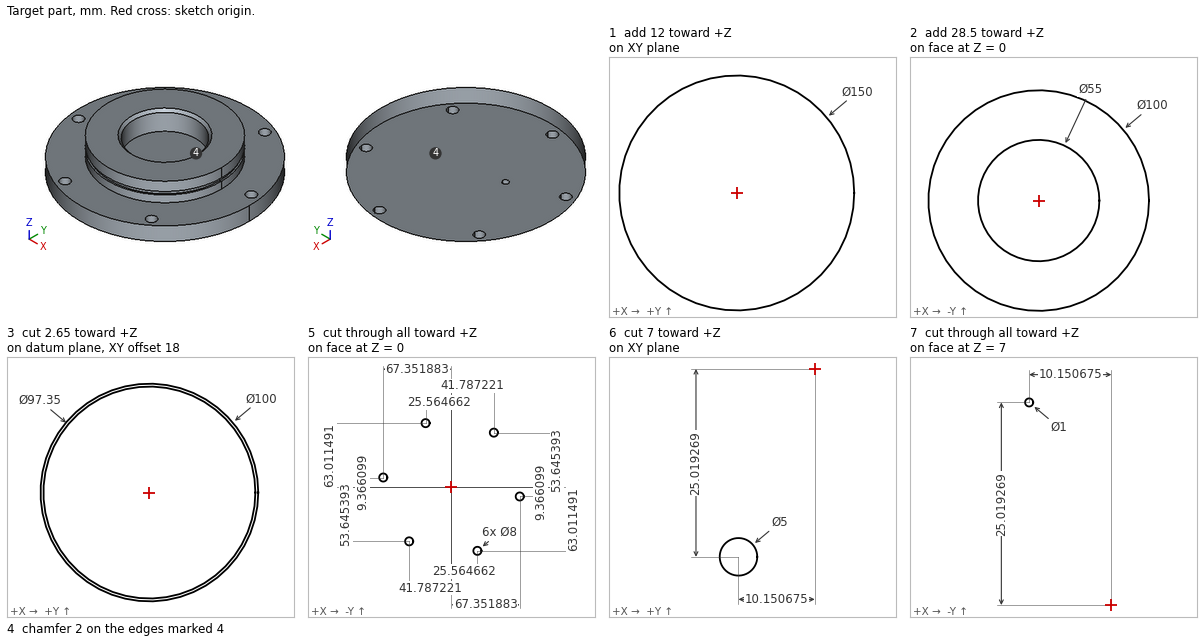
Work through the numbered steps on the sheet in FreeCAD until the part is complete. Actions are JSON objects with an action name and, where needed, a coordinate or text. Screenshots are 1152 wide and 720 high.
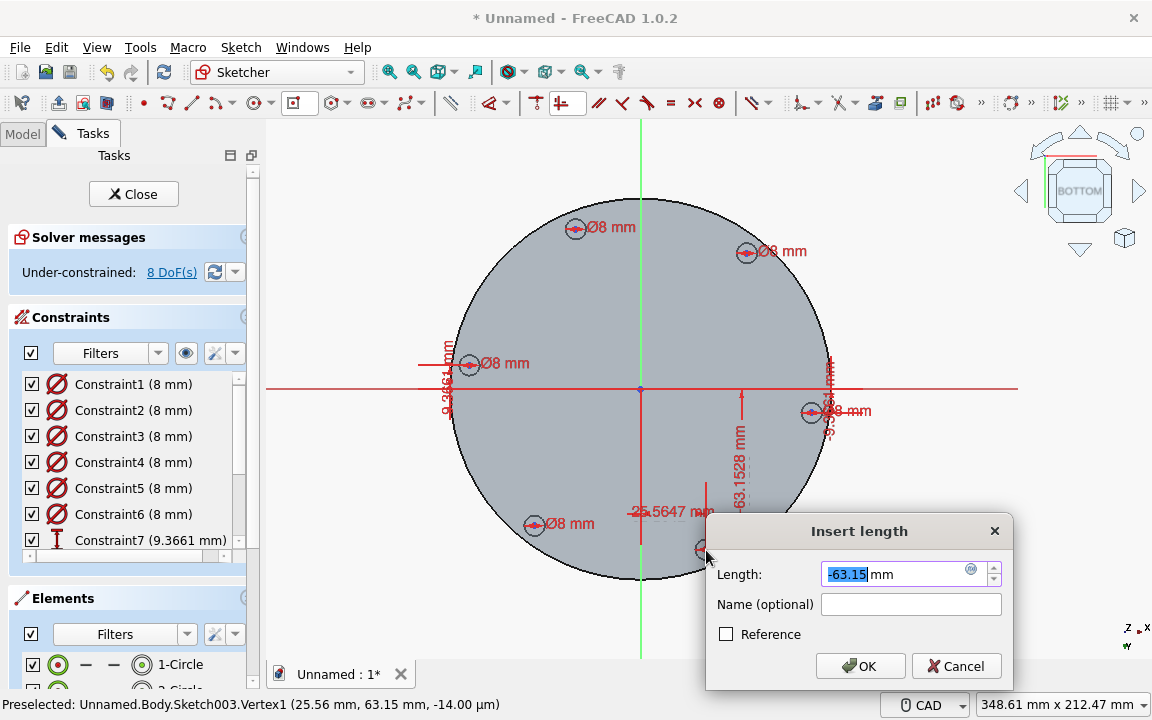
{"action": "type", "text": "-63.011491"}
{"action": "key", "text": "Return"}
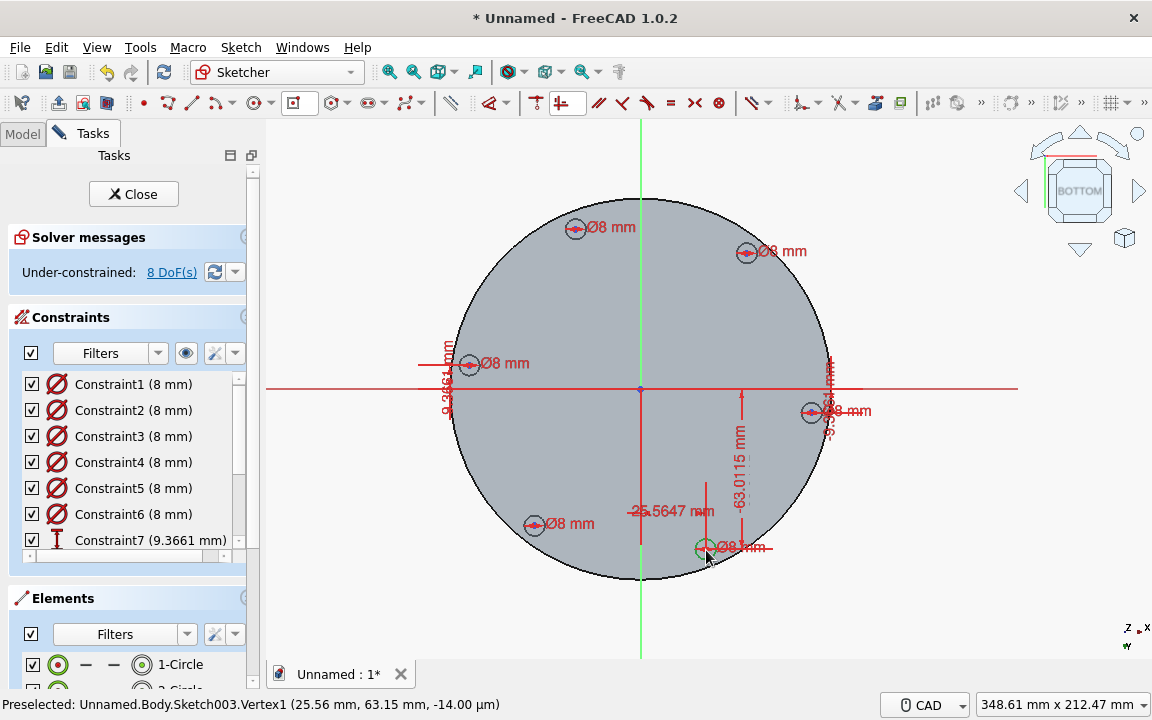
{"action": "left_click", "coordinate": [535, 526]}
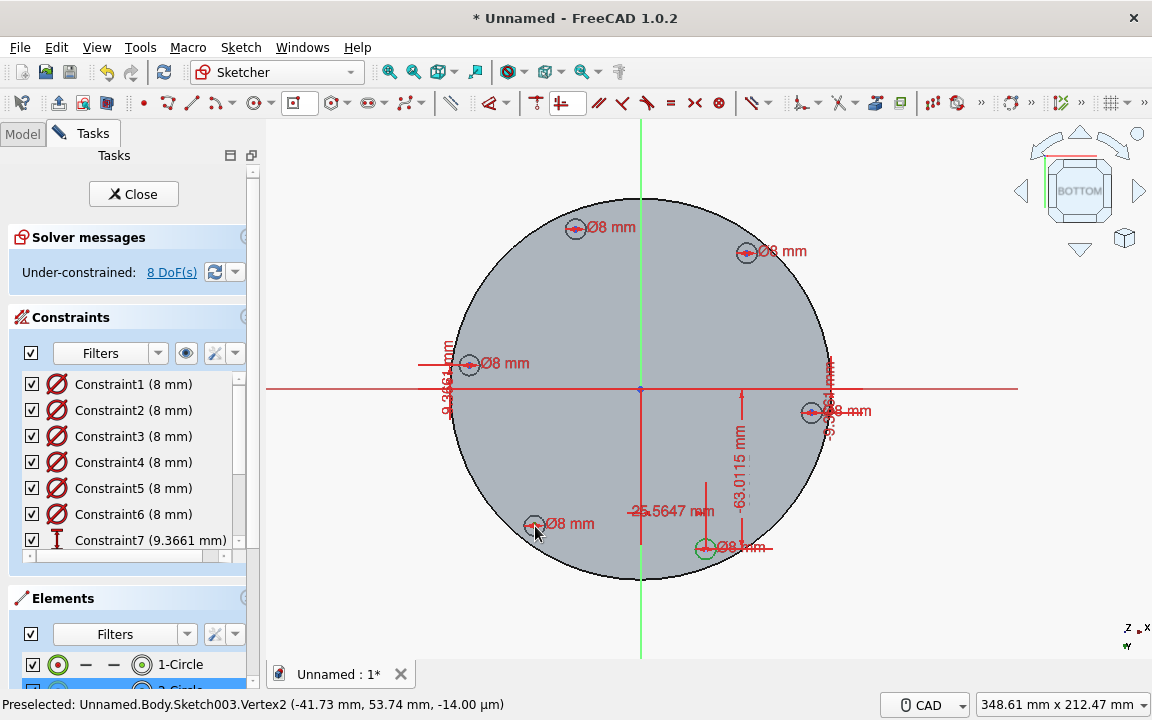
{"action": "left_click", "coordinate": [508, 104]}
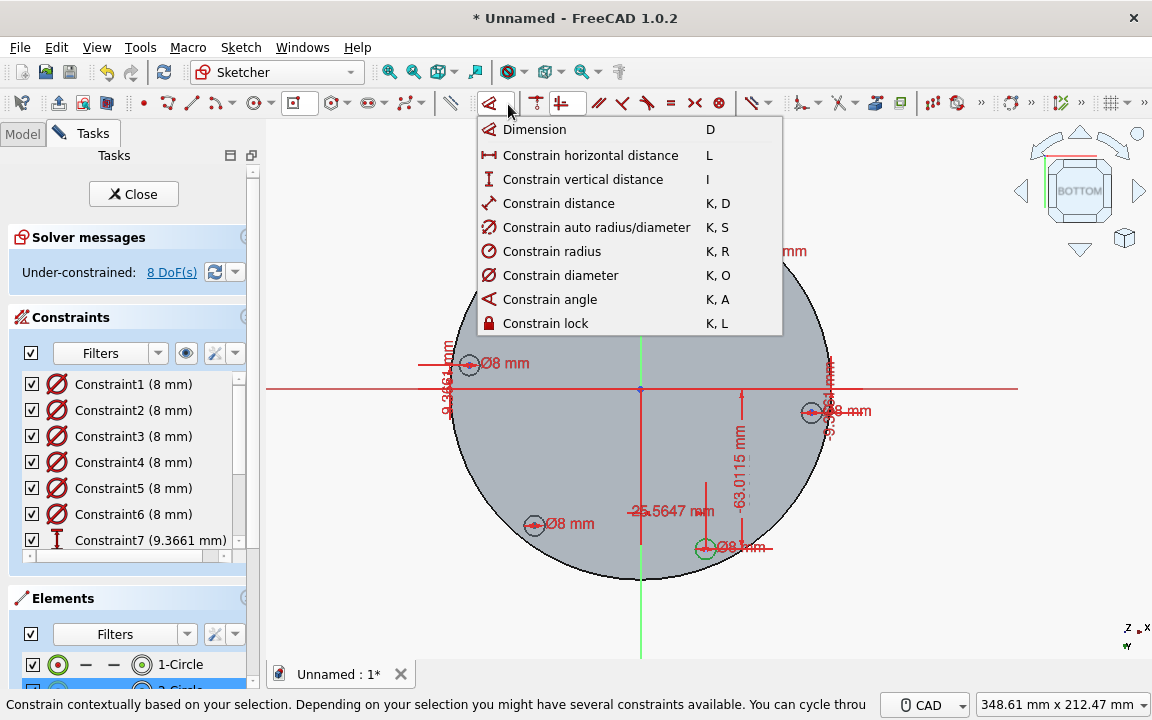
{"action": "left_click", "coordinate": [630, 155]}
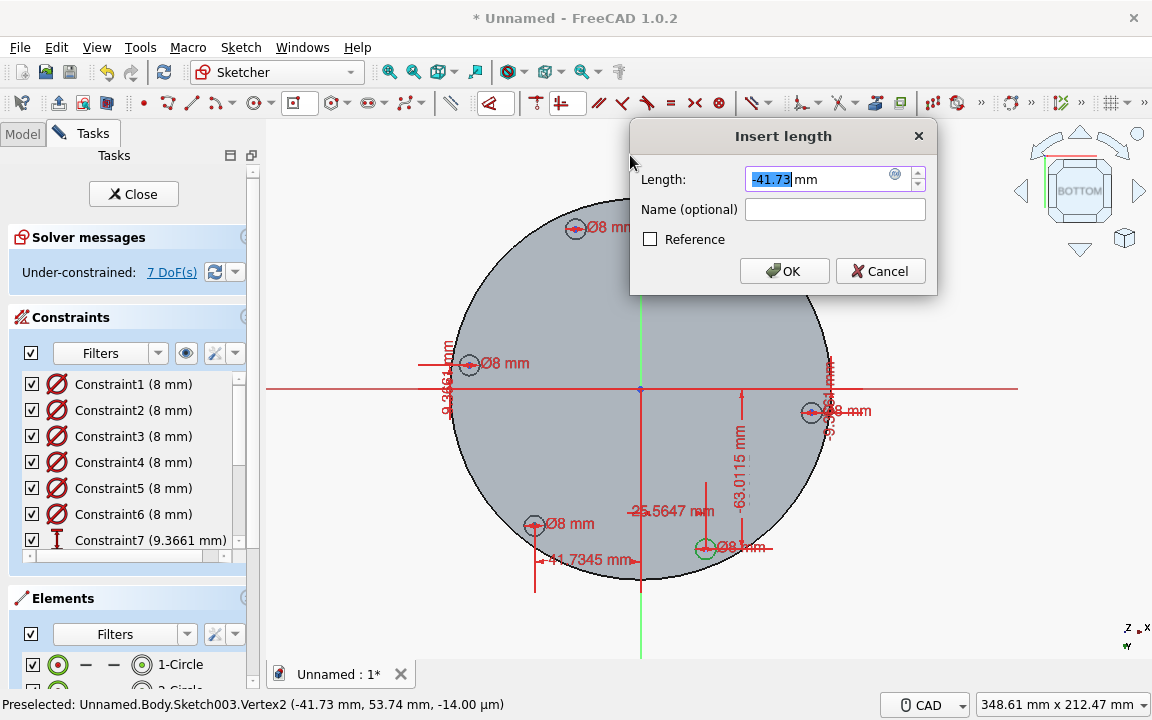
{"action": "type", "text": "-41.787221"}
{"action": "key", "text": "Return"}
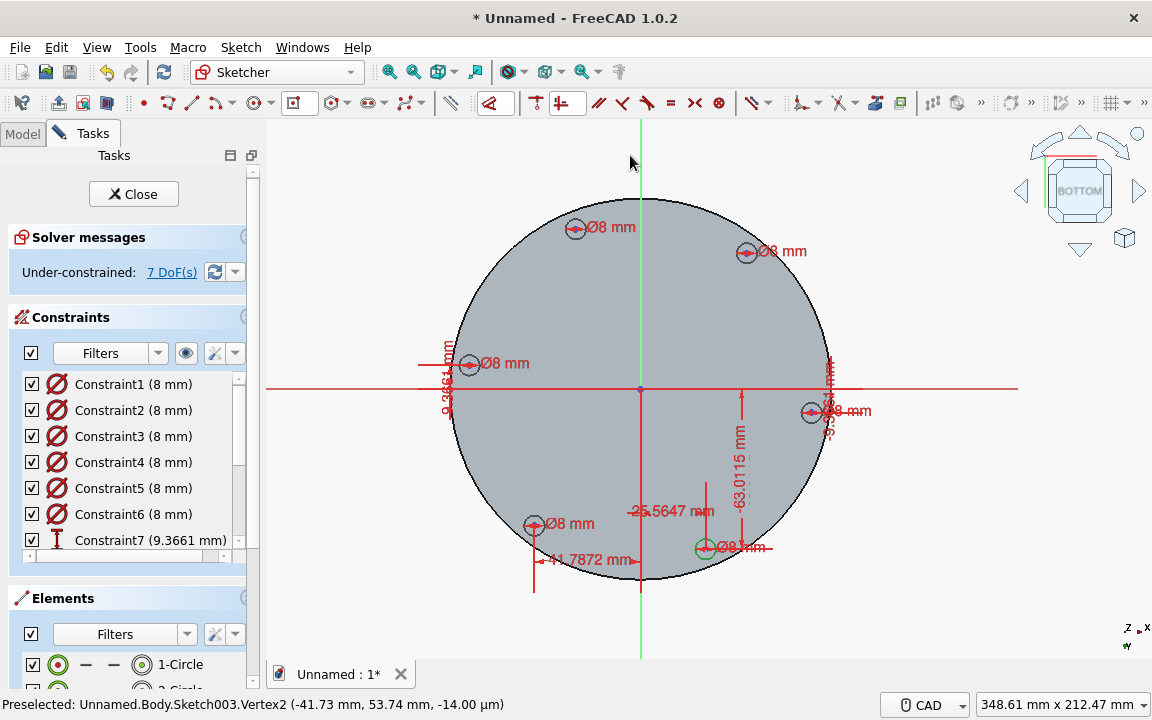
{"action": "left_click", "coordinate": [534, 526]}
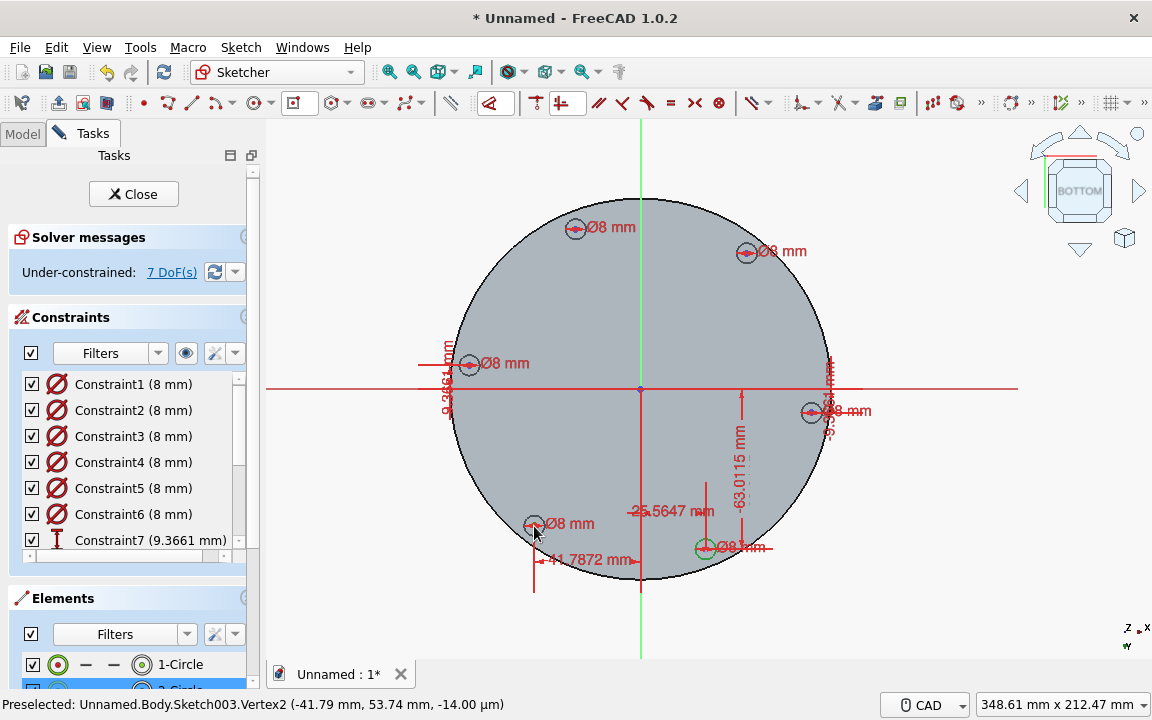
{"action": "key", "text": "i"}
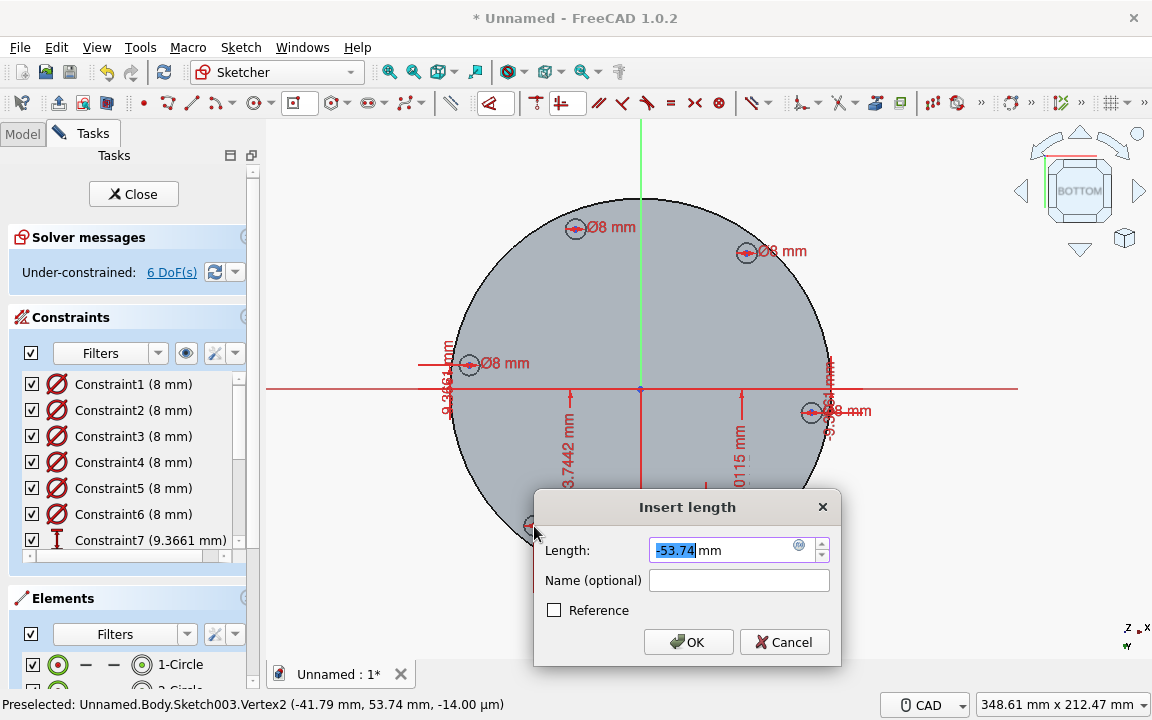
{"action": "type", "text": "-53.645393"}
{"action": "key", "text": "Return"}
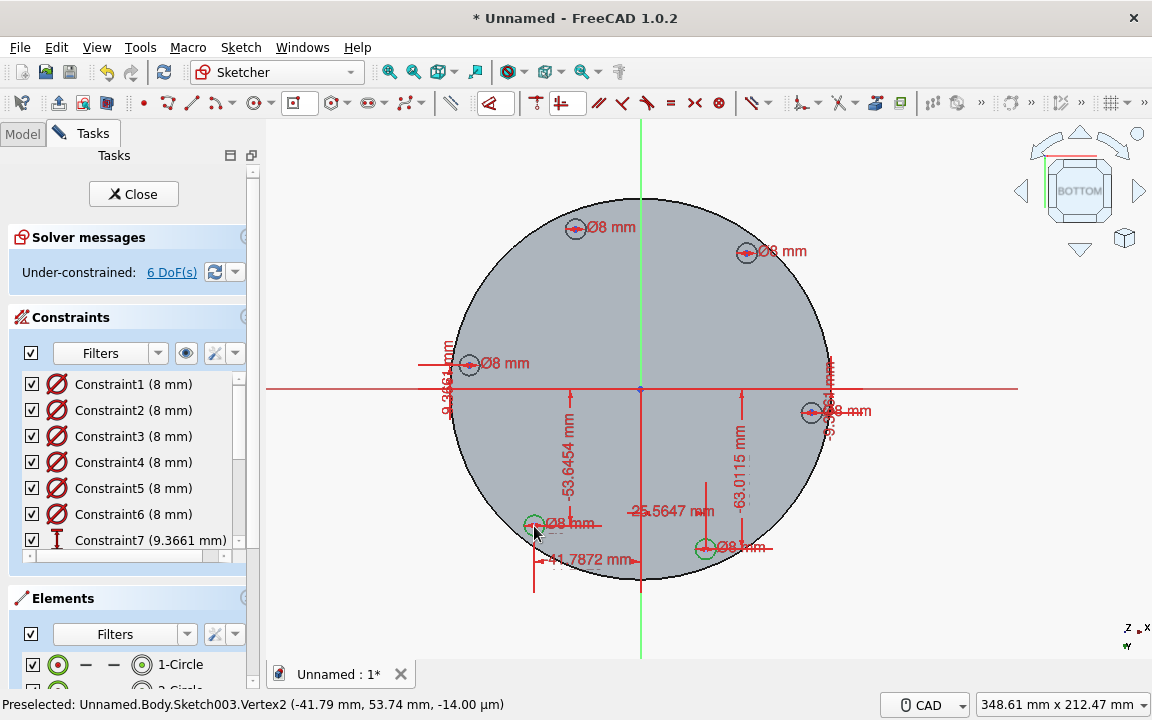
{"action": "left_click", "coordinate": [470, 365]}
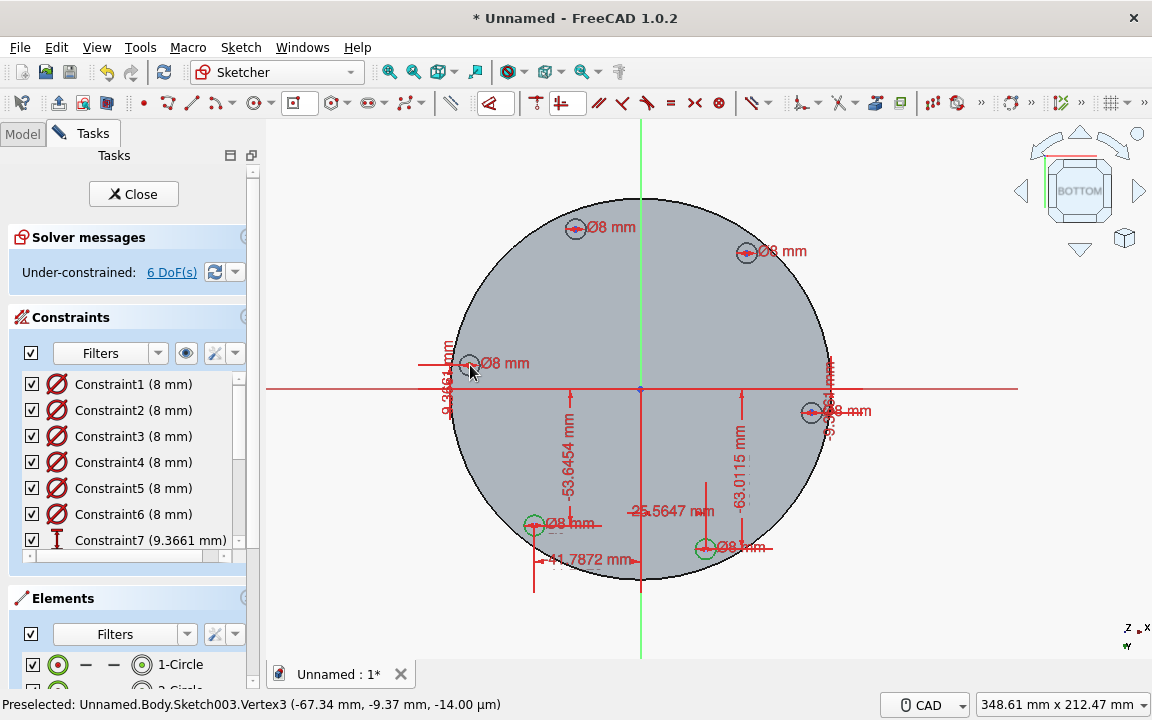
{"action": "left_click", "coordinate": [508, 104]}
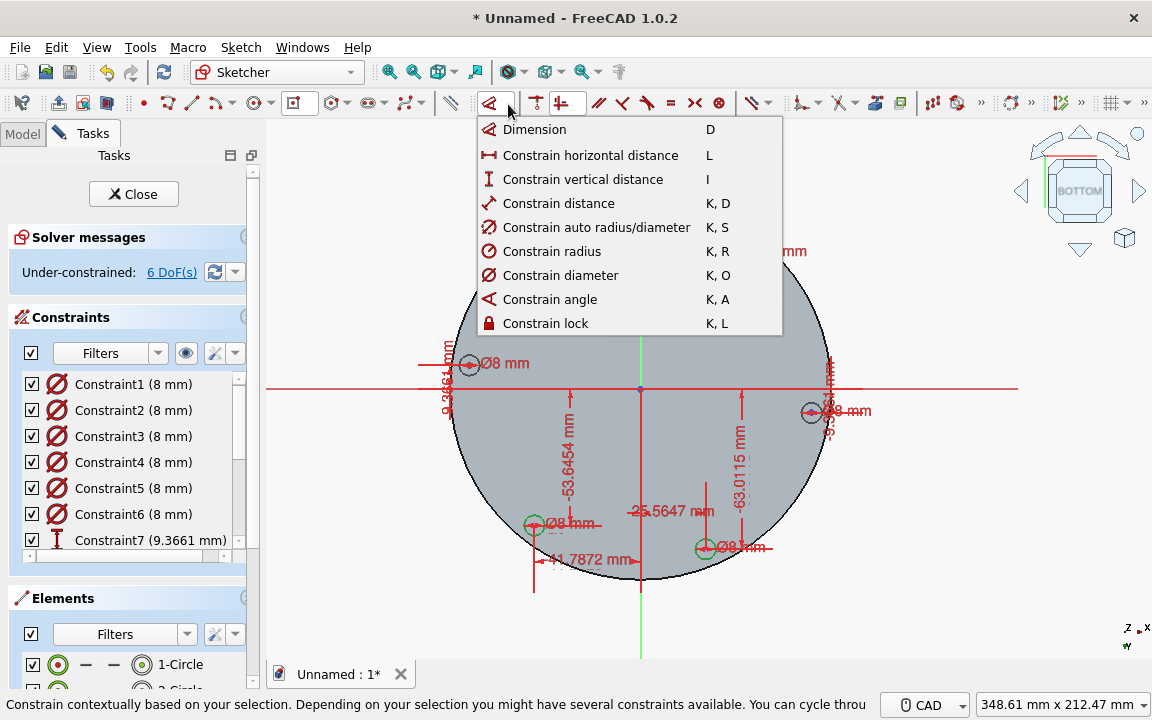
{"action": "left_click", "coordinate": [630, 155]}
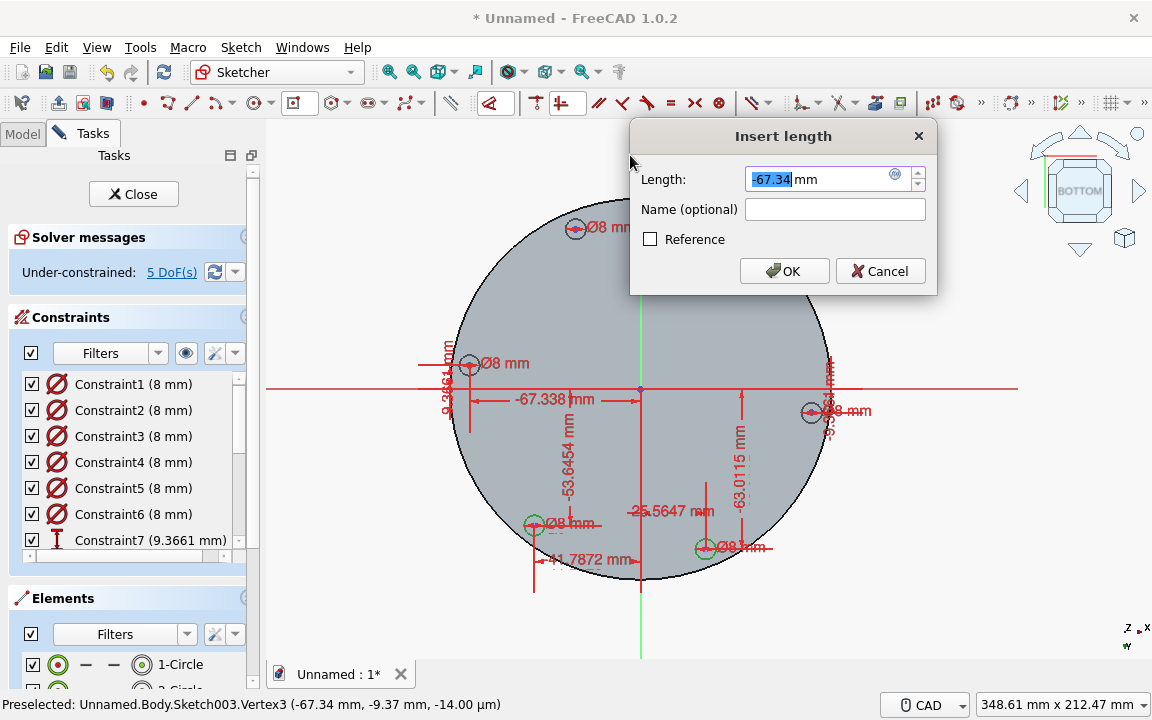
{"action": "type", "text": "-67.351883"}
{"action": "key", "text": "Return"}